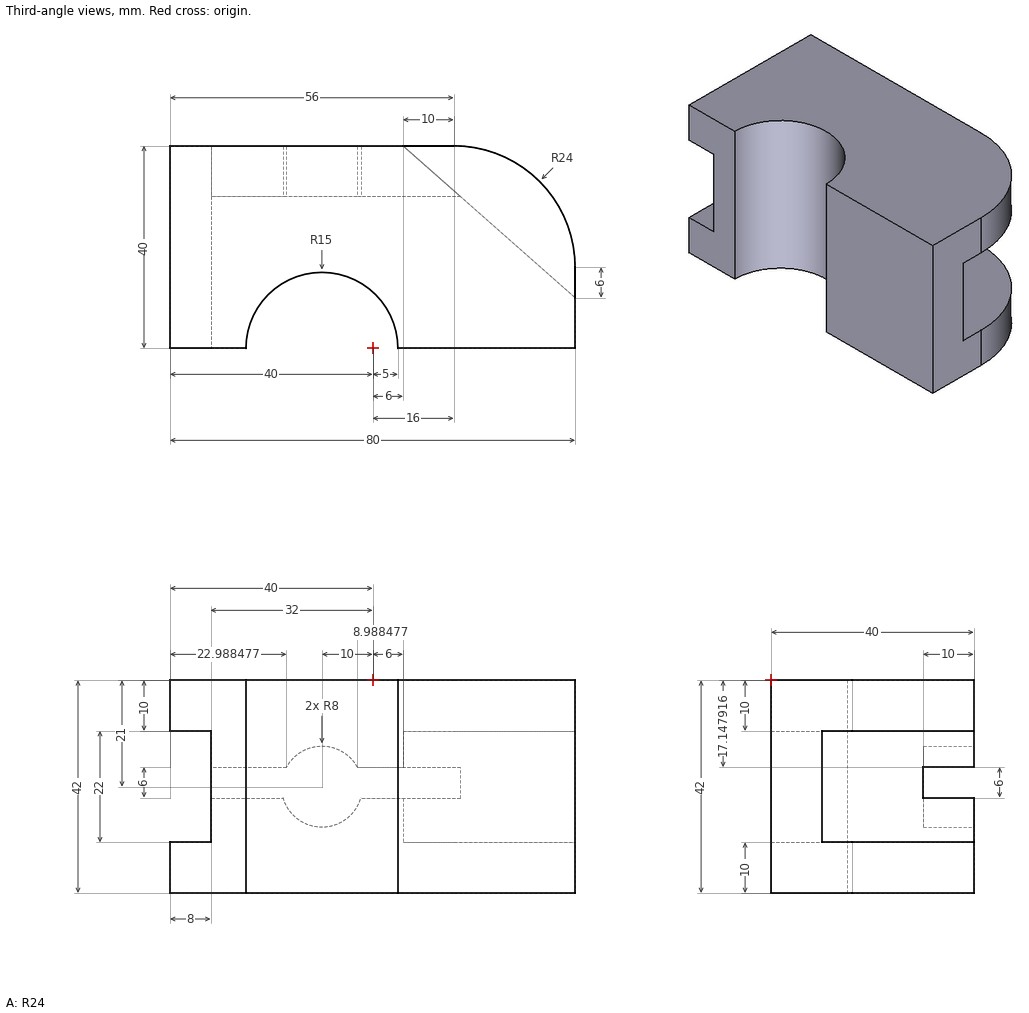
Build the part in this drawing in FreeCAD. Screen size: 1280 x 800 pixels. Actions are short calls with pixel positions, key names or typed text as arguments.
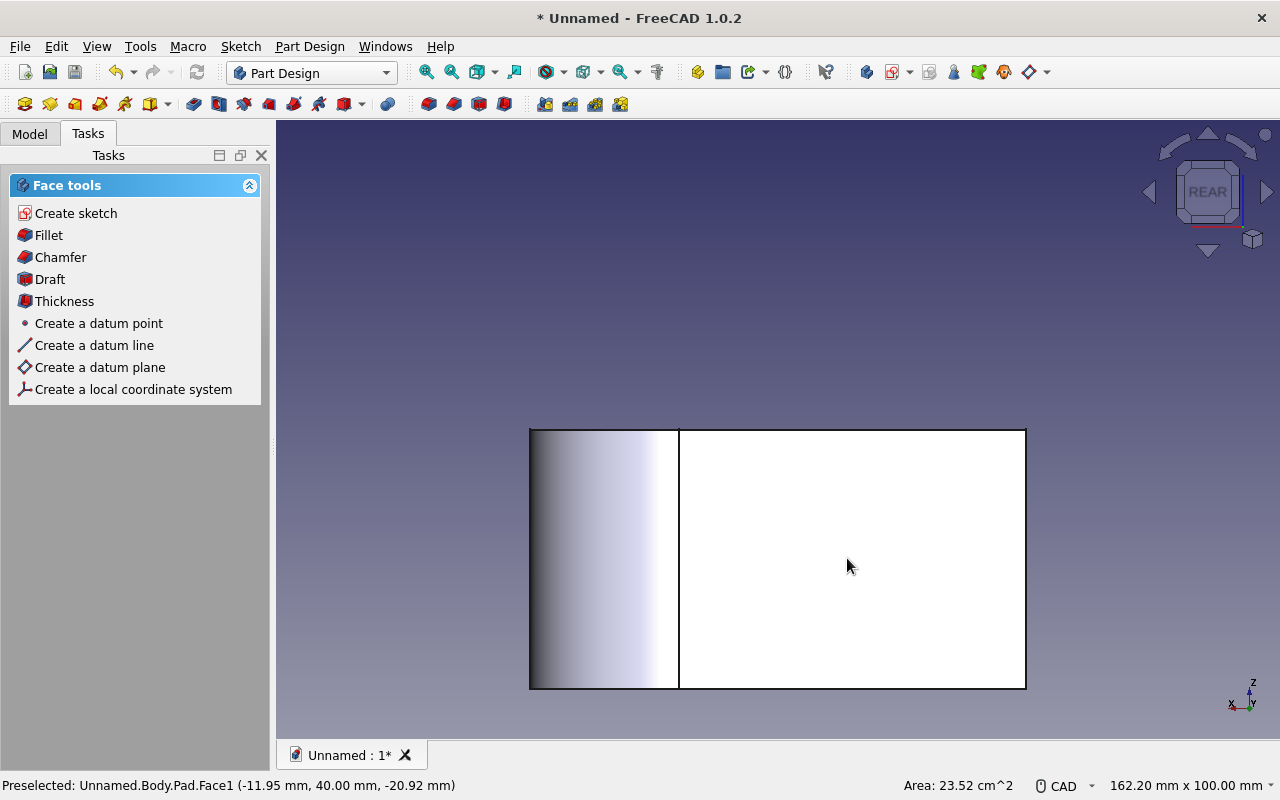
click(892, 72)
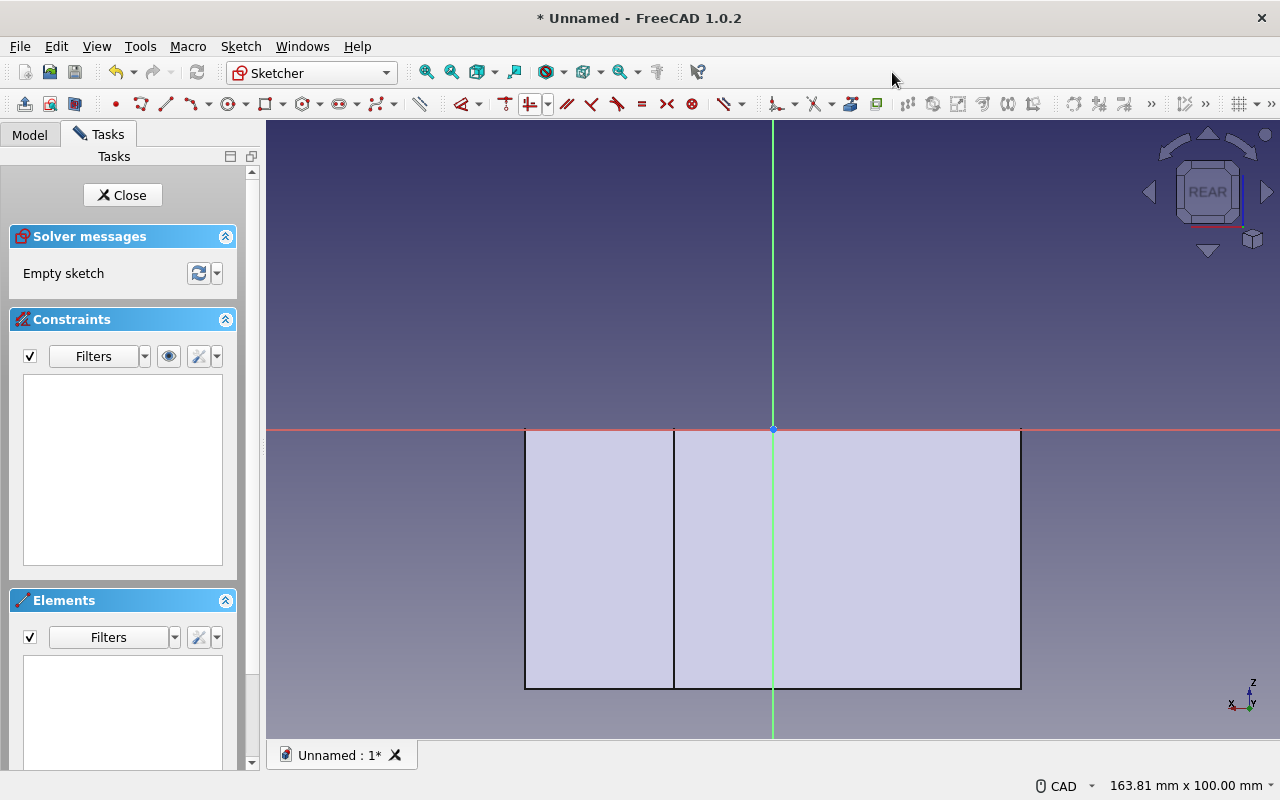
scroll(1020, 592, up, 4)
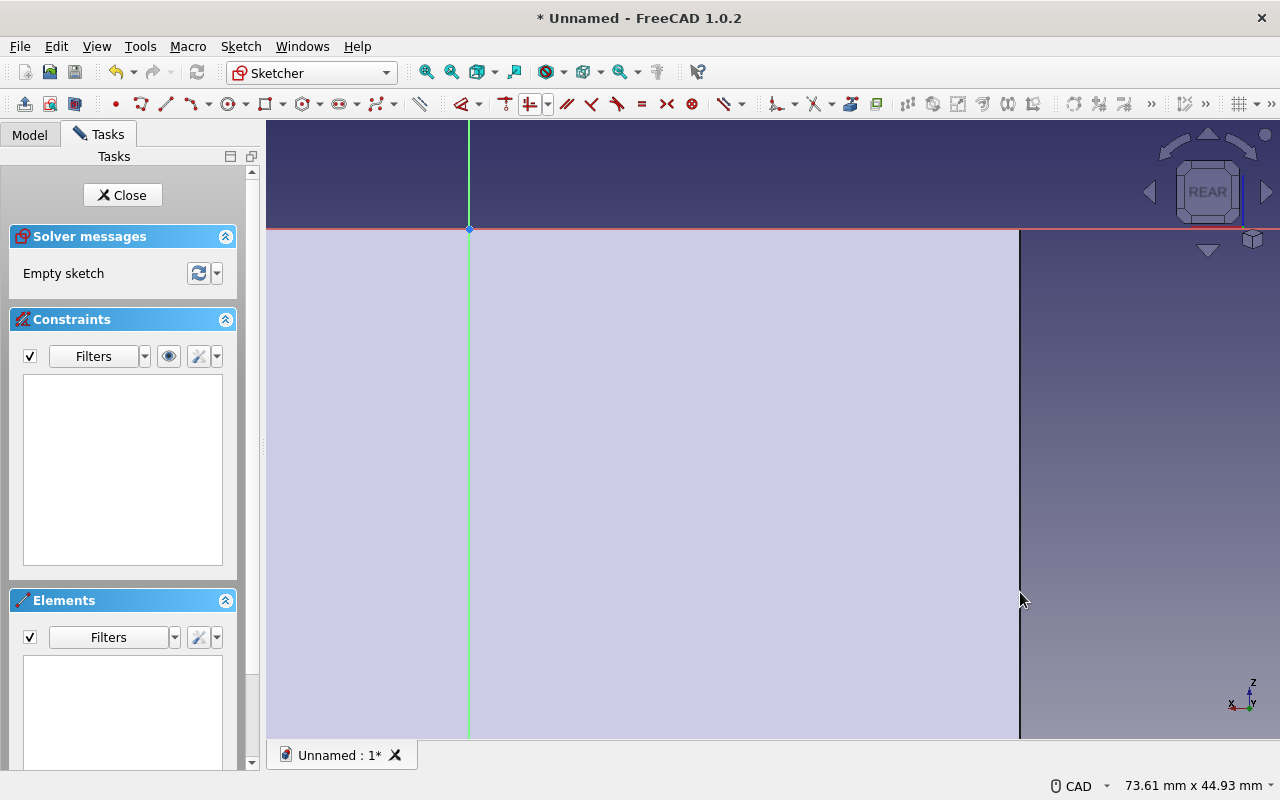
key(g)
key(m)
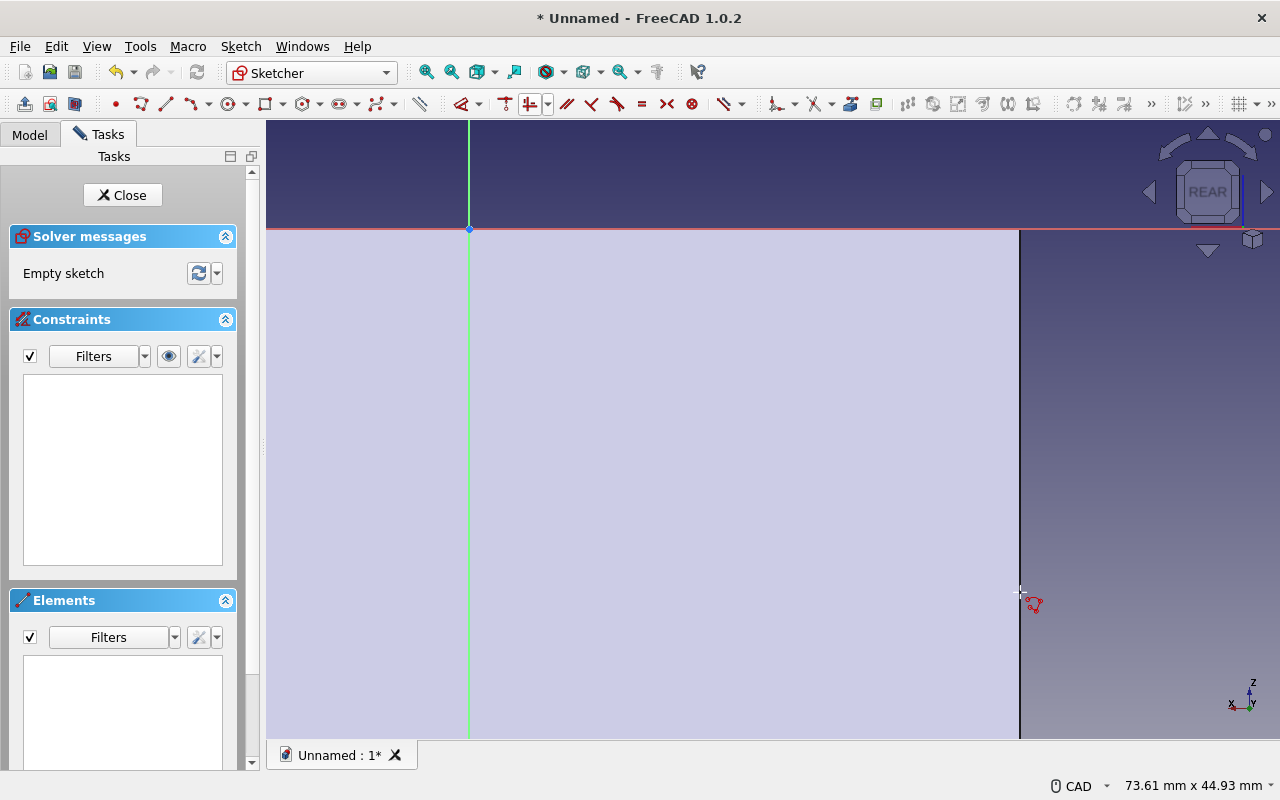
click(713, 548)
click(1020, 548)
click(1020, 466)
click(704, 466)
right_click(704, 466)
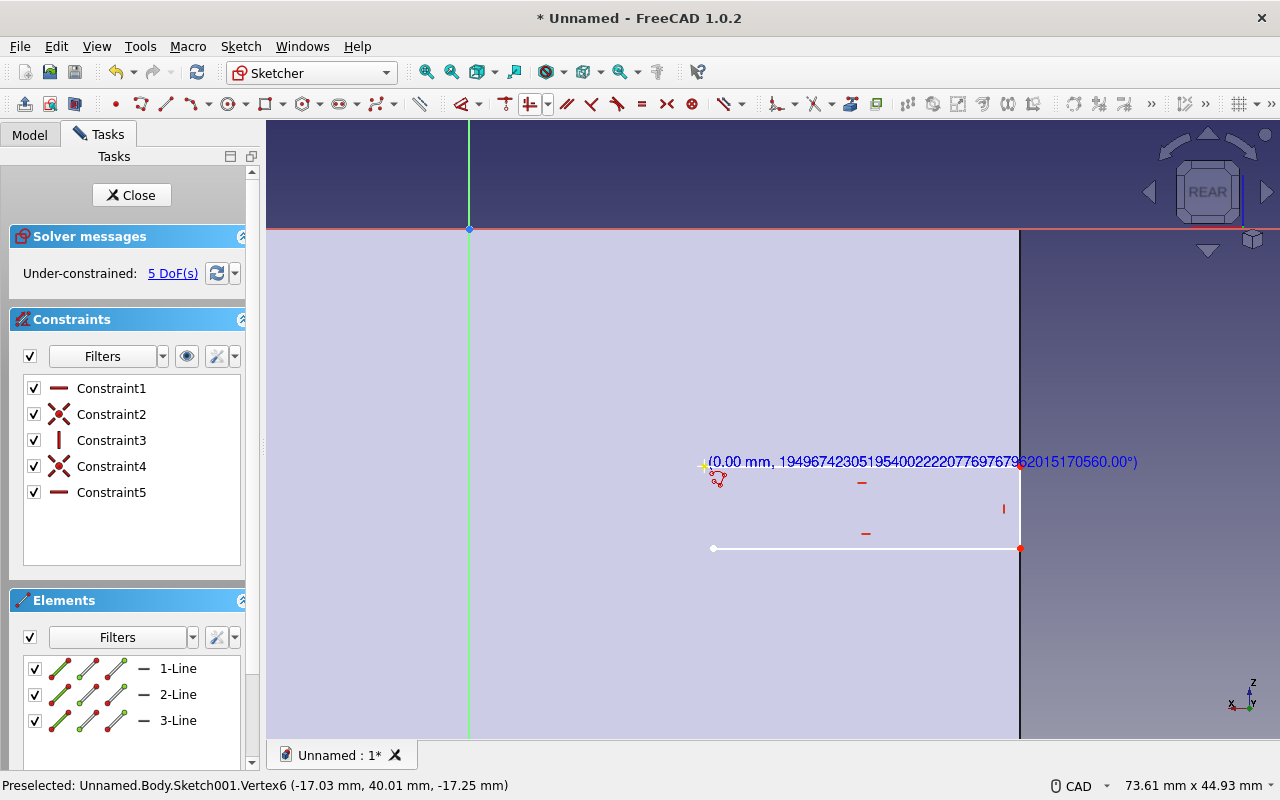
click(511, 466)
click(387, 466)
click(387, 548)
click(501, 548)
right_click(501, 548)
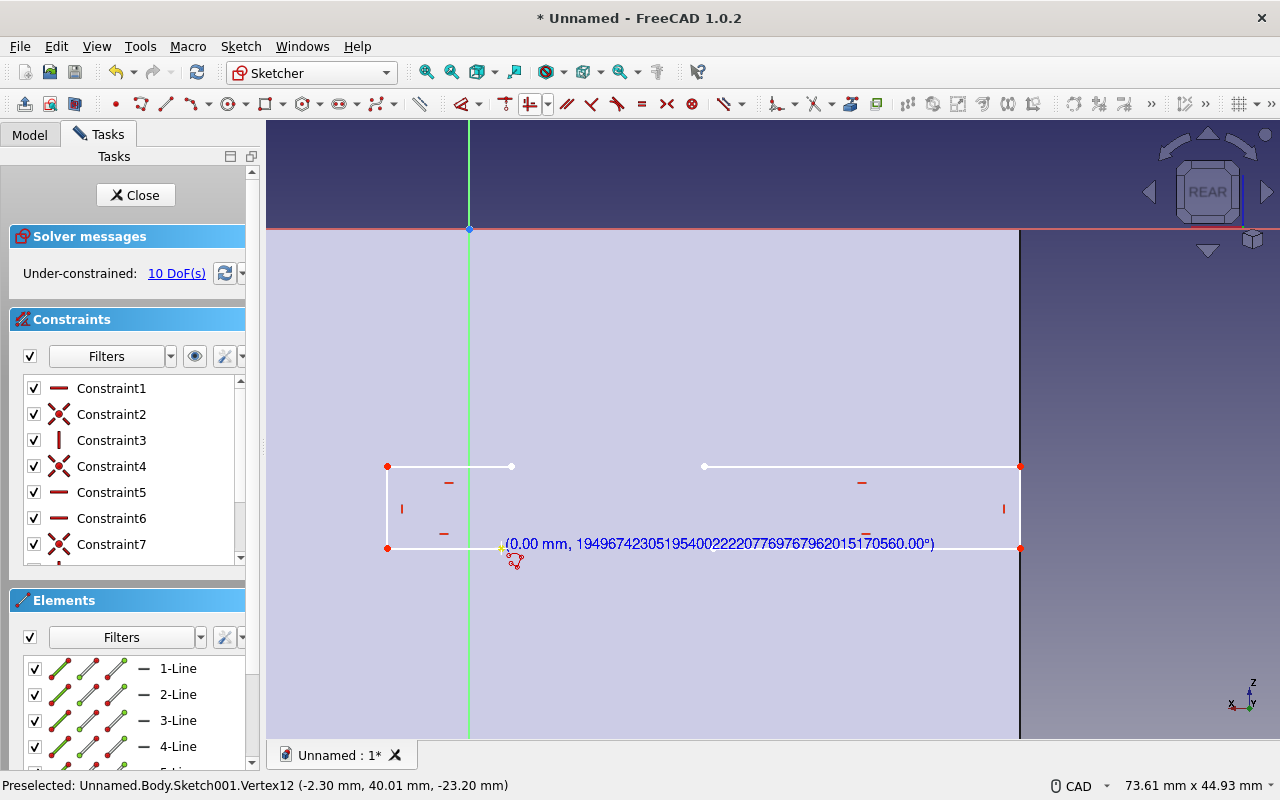
key(g)
key(3)
key(a)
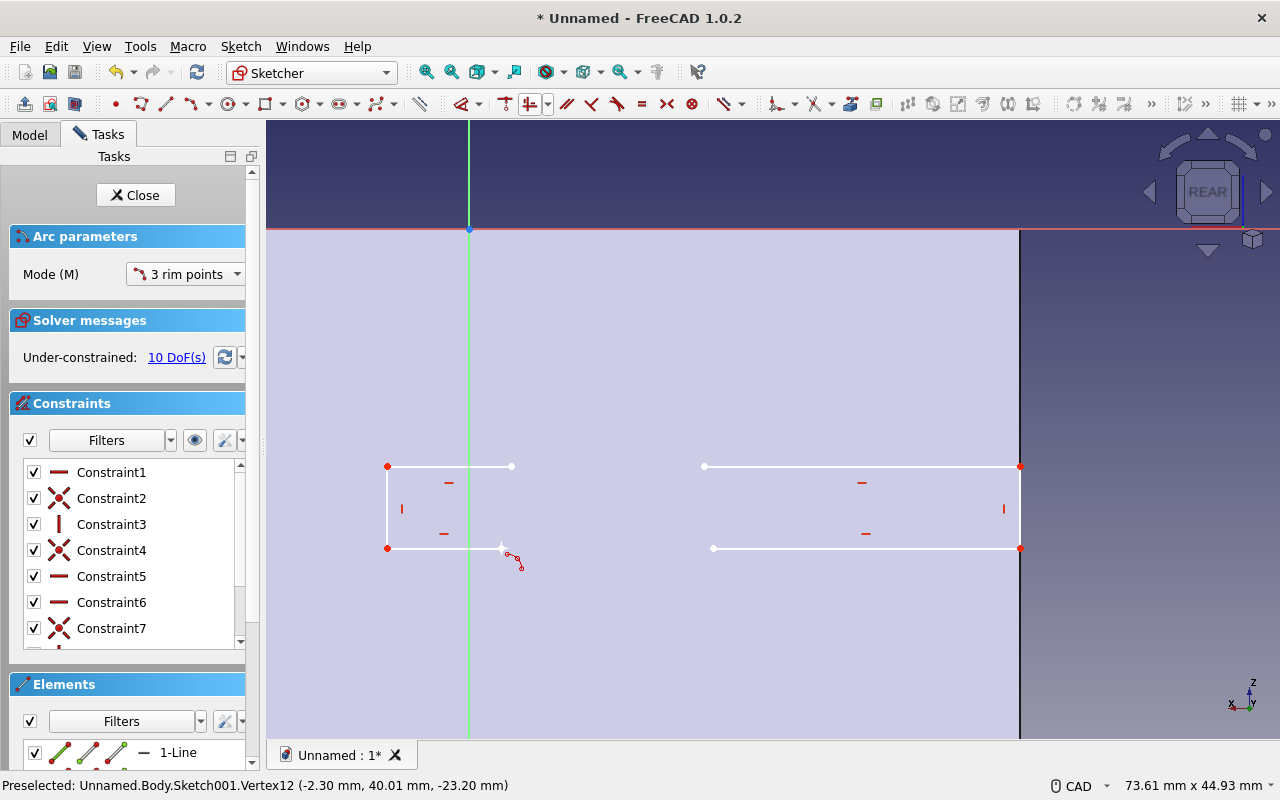
click(704, 467)
click(511, 467)
click(607, 409)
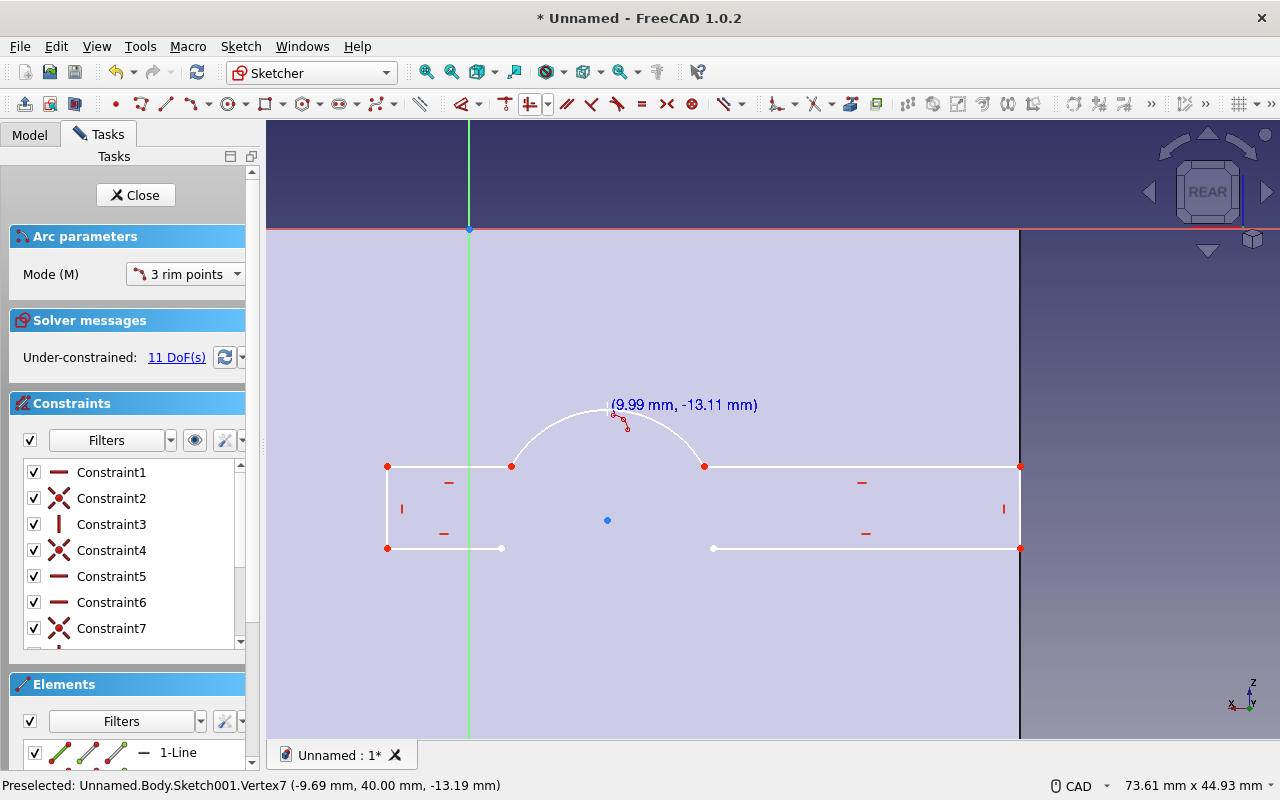
click(501, 549)
click(713, 549)
click(607, 629)
key(Escape)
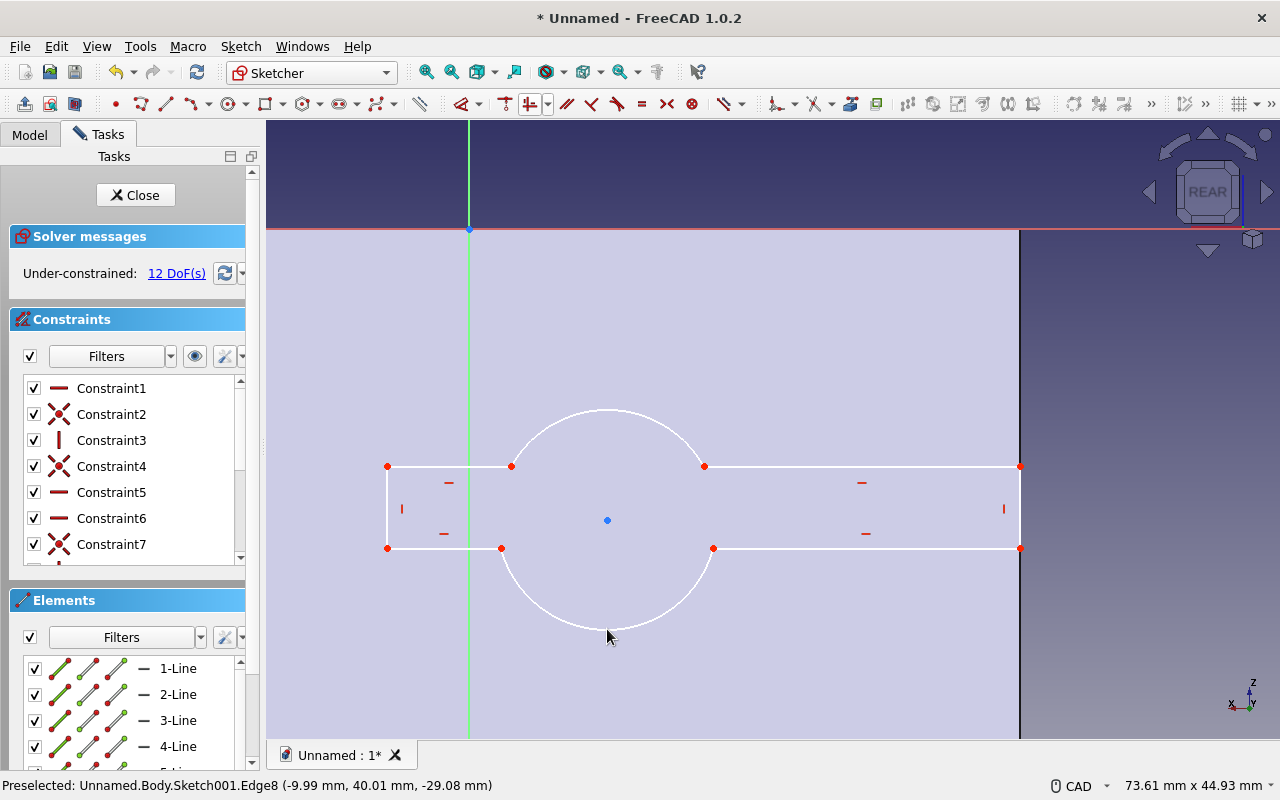
click(653, 420)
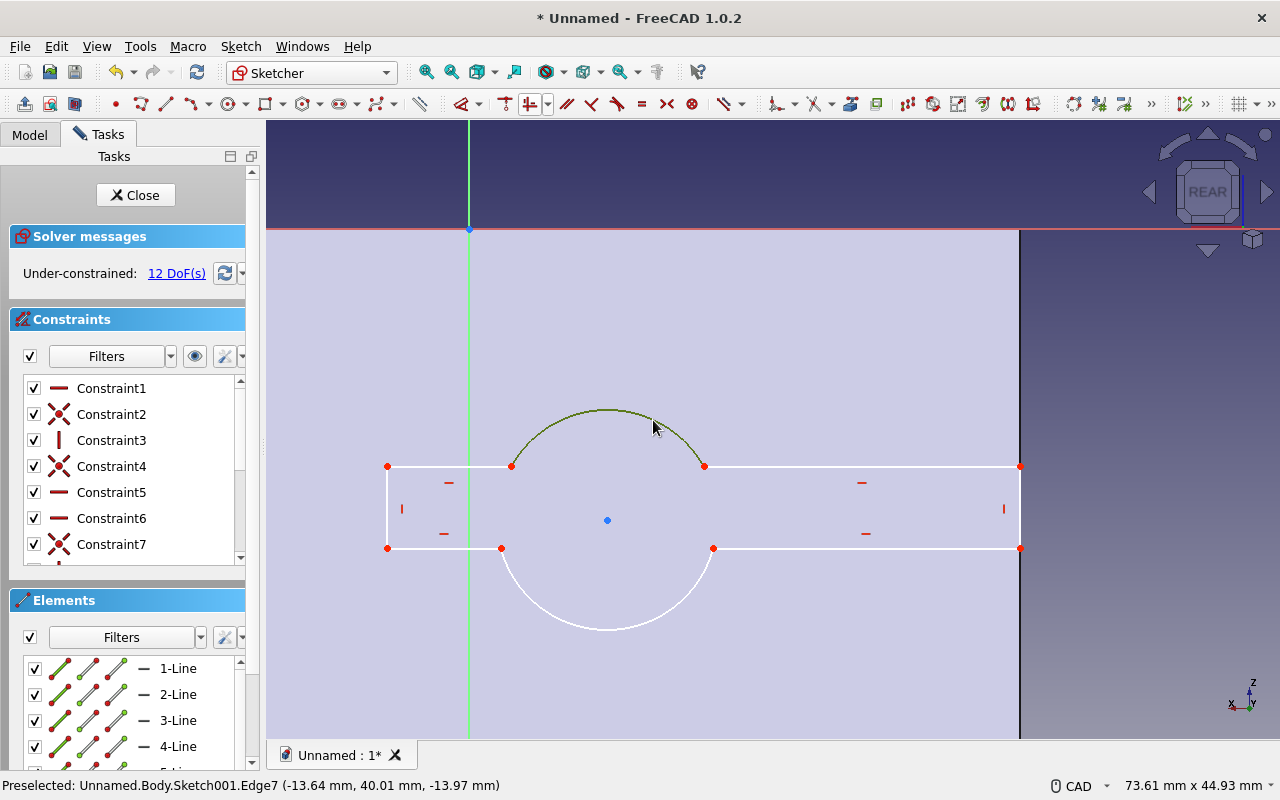
click(552, 615)